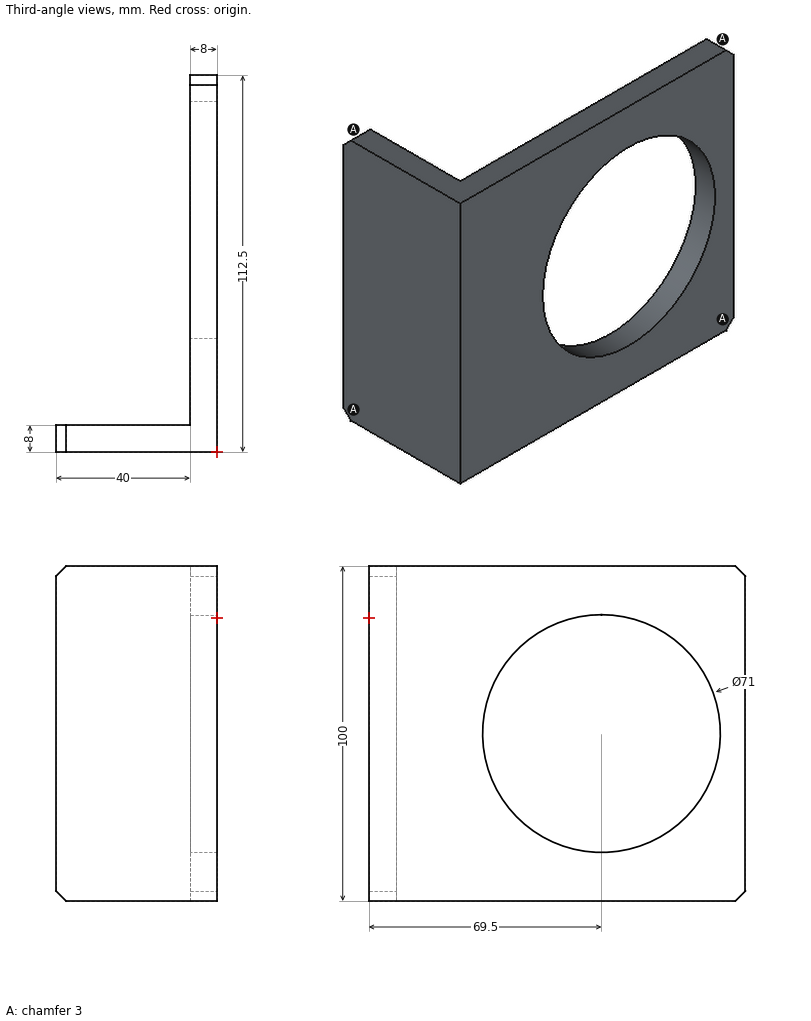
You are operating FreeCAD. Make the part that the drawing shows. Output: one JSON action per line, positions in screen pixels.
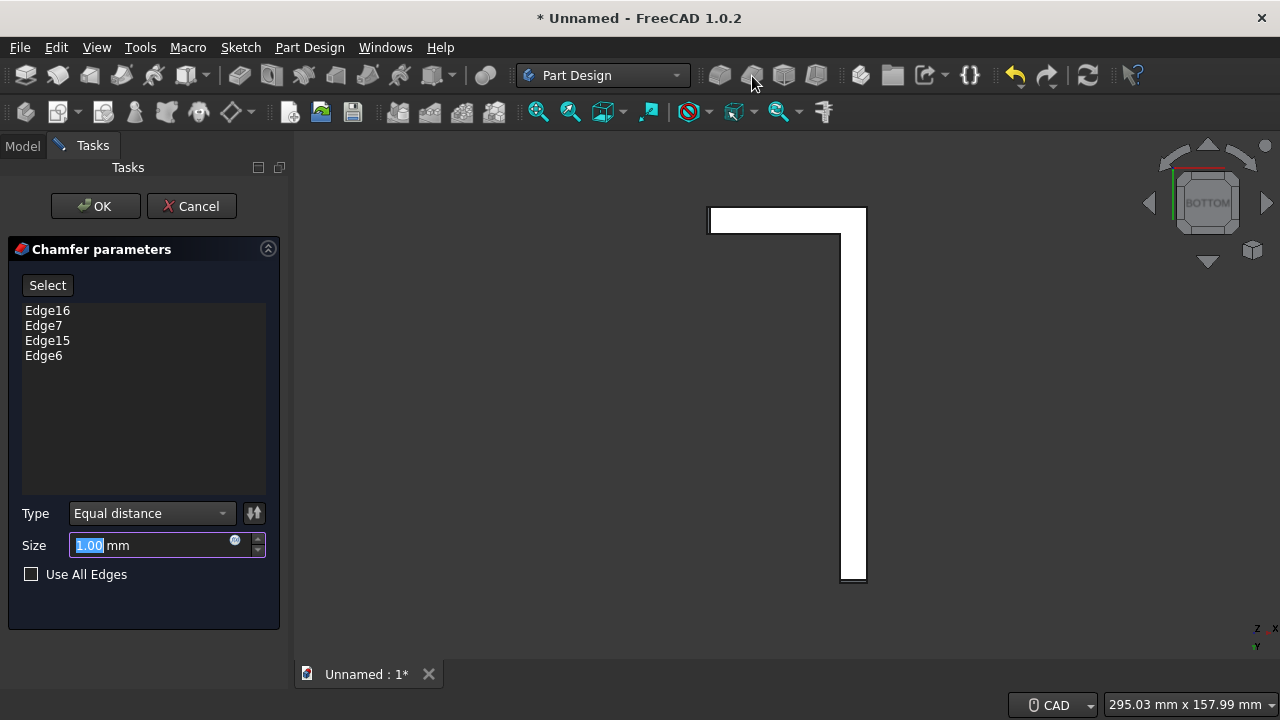
{"action": "type", "text": "3"}
{"action": "key", "text": "Tab"}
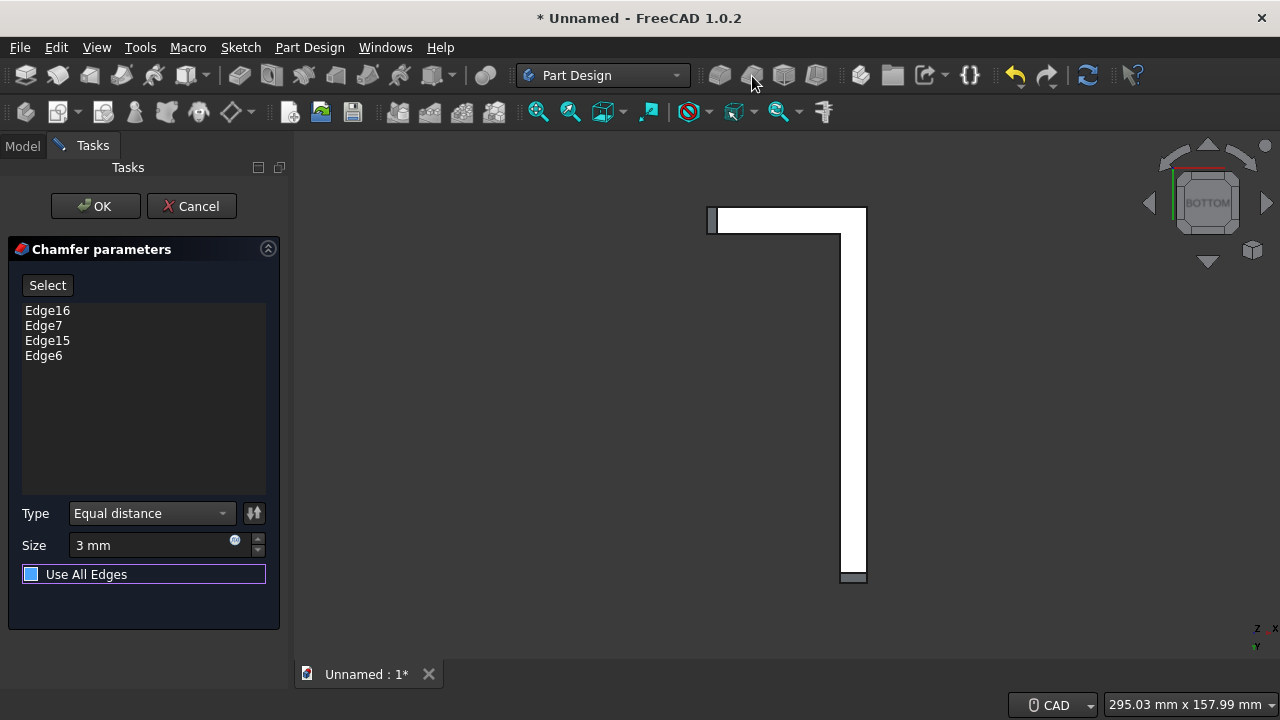
{"action": "left_click", "coordinate": [96, 206]}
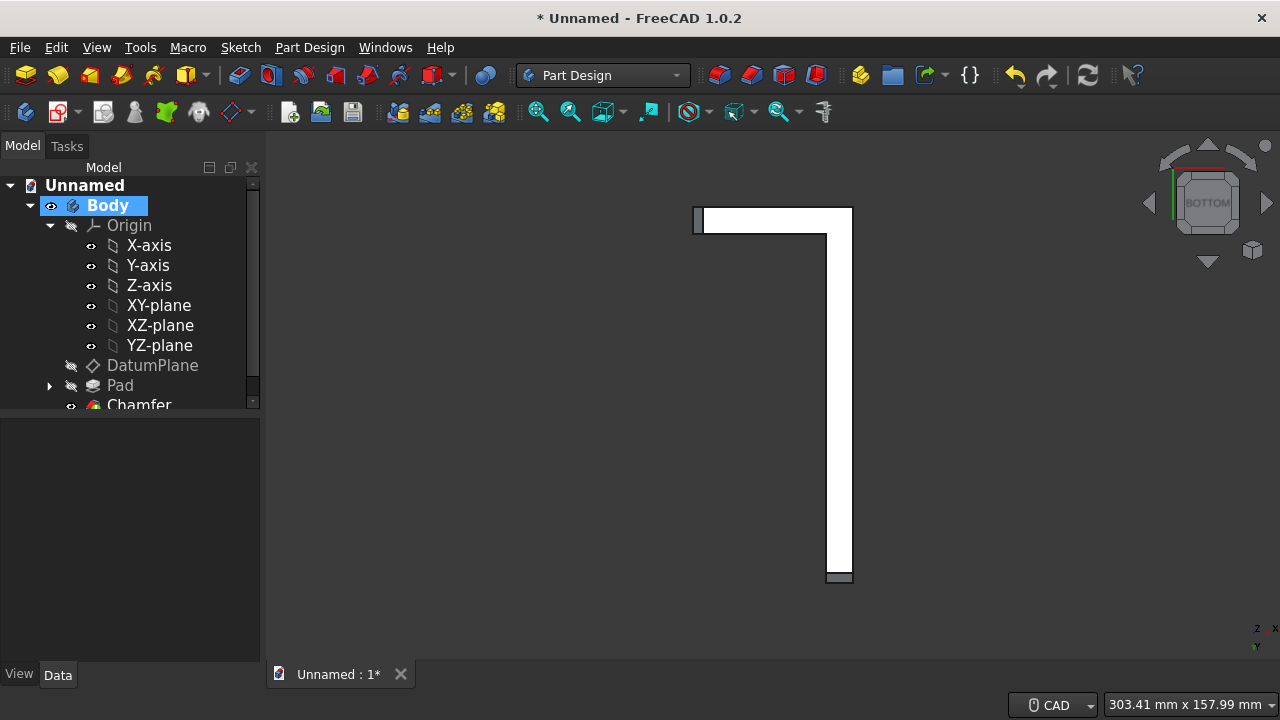
{"action": "key", "text": "6"}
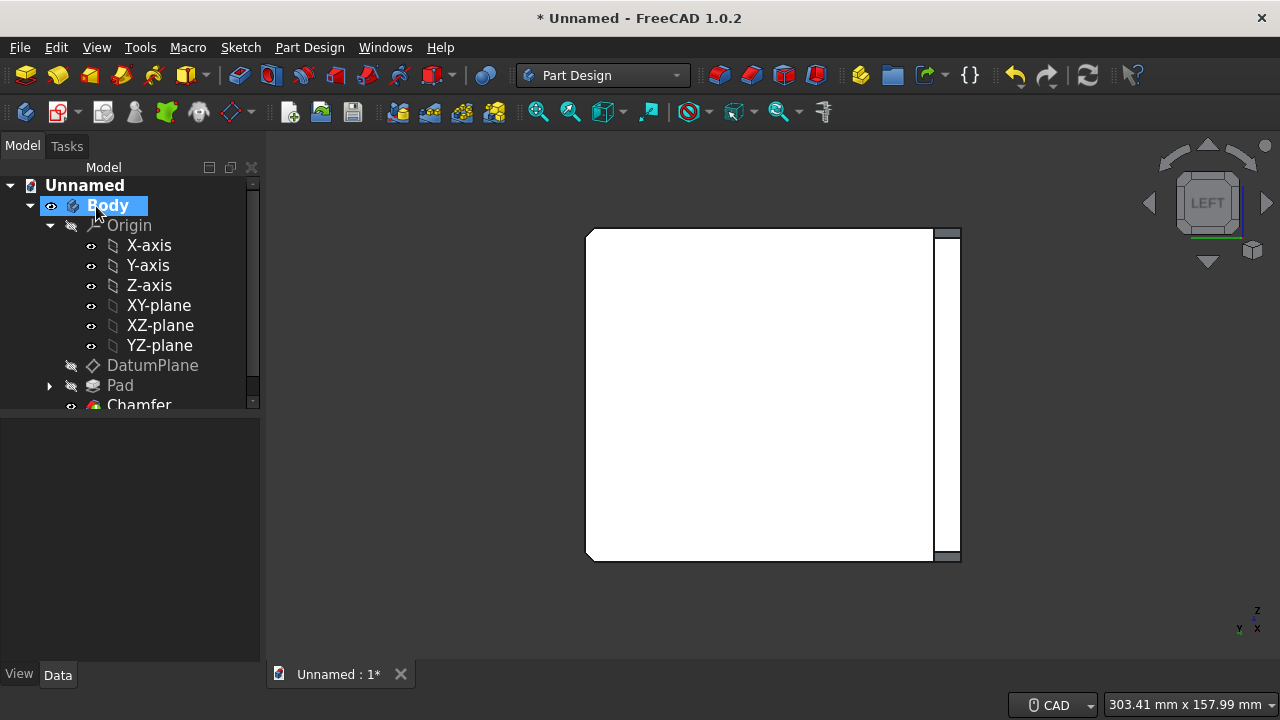
{"action": "left_click", "coordinate": [760, 394]}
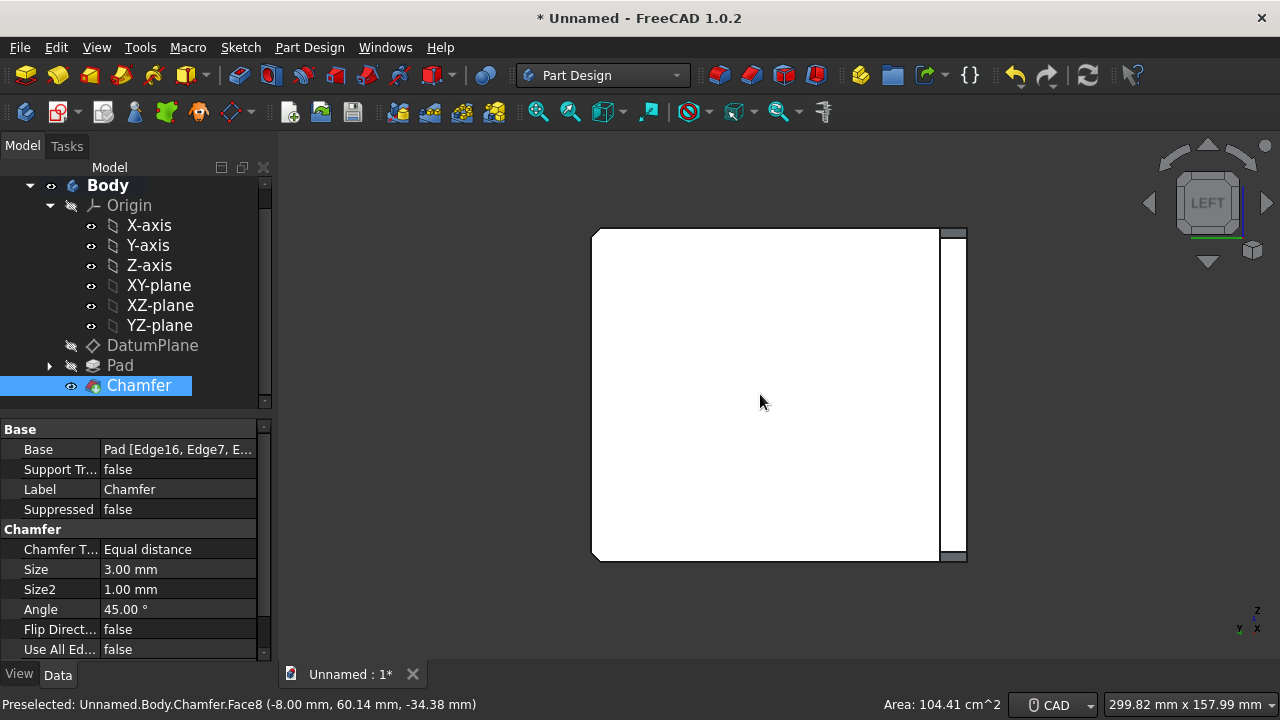
{"action": "left_click", "coordinate": [58, 112]}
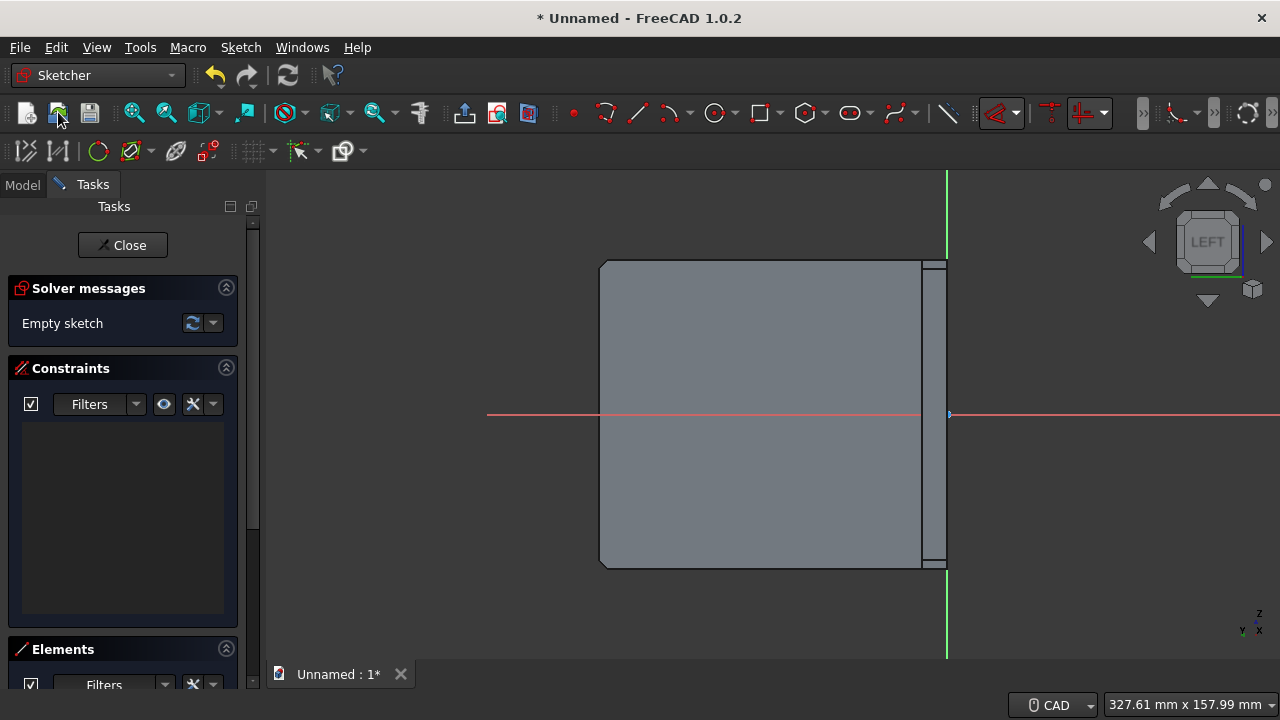
{"action": "left_click", "coordinate": [530, 114]}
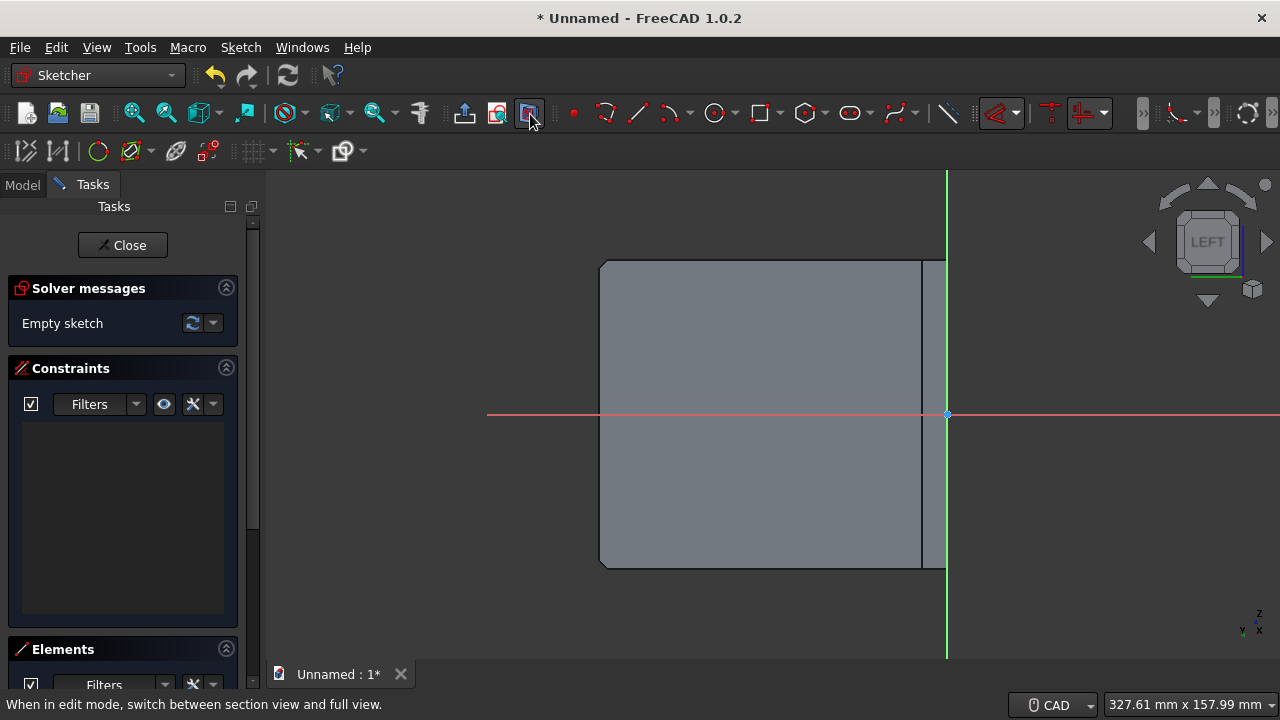
{"action": "scroll", "coordinate": [947, 414], "scroll_direction": "up", "scroll_amount": 2}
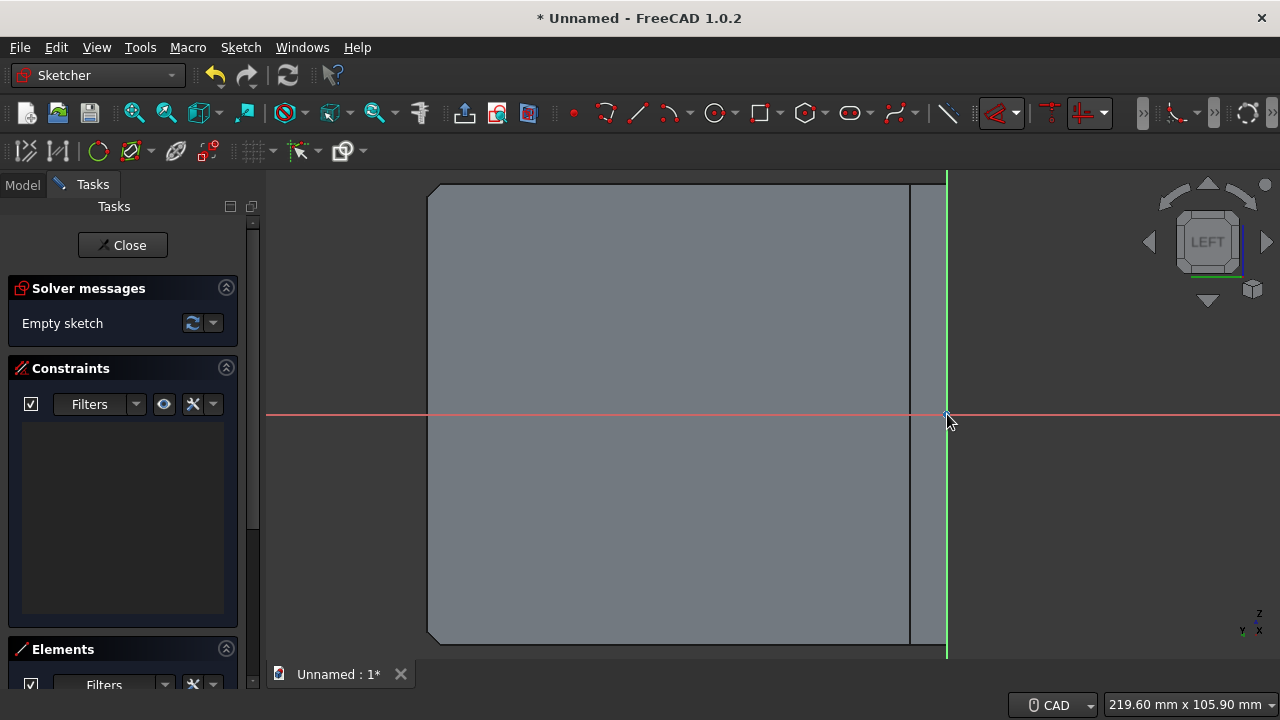
{"action": "left_click", "coordinate": [716, 114]}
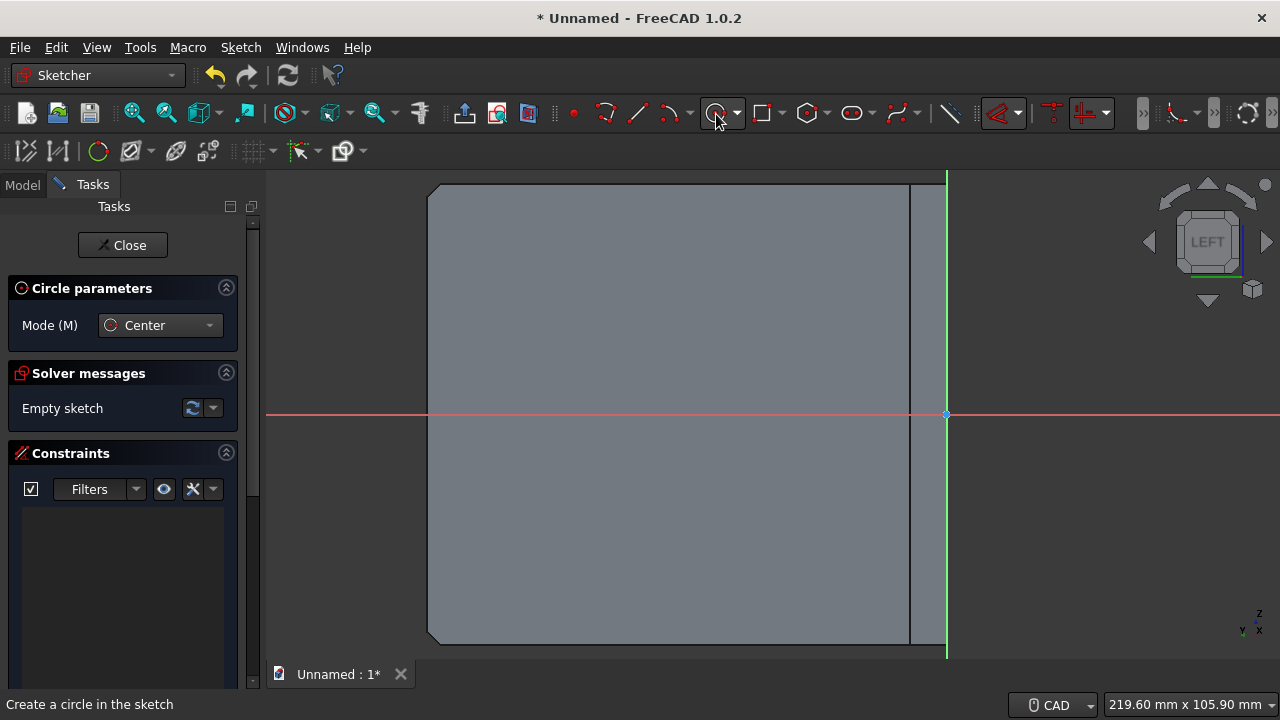
{"action": "left_click", "coordinate": [626, 414]}
{"action": "left_click", "coordinate": [742, 299]}
{"action": "key", "text": "Escape"}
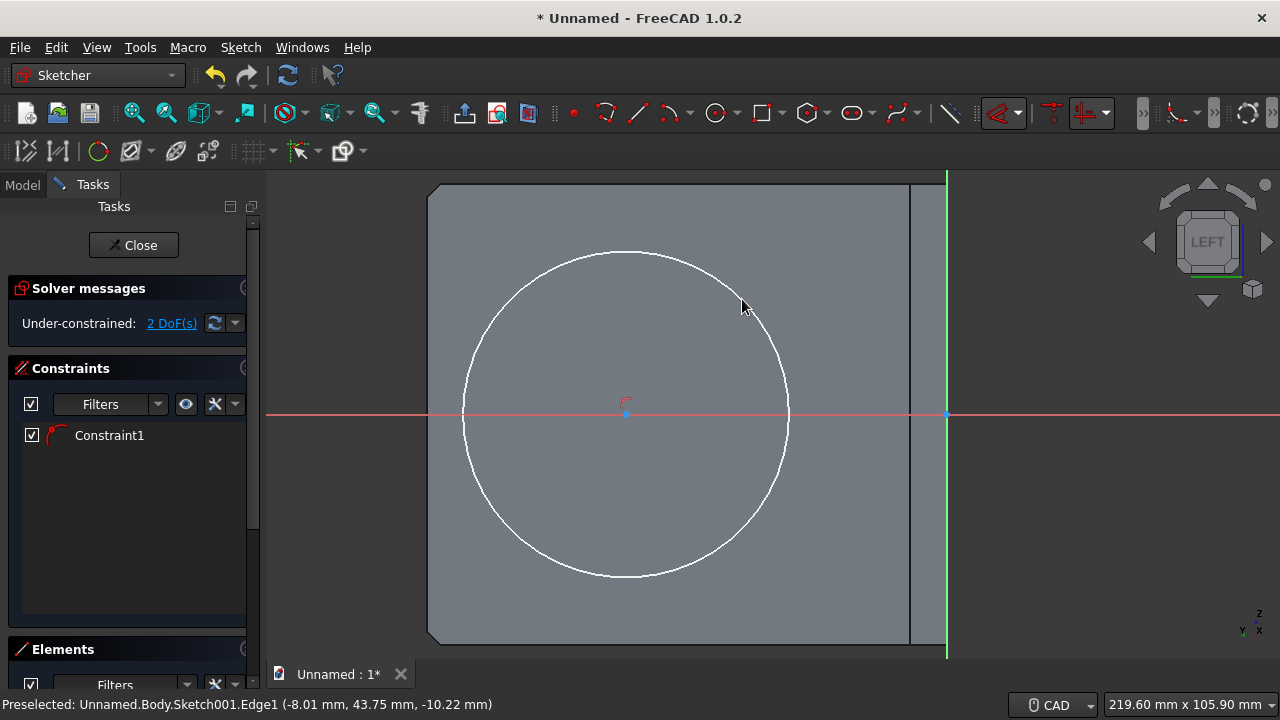
{"action": "left_click", "coordinate": [741, 299]}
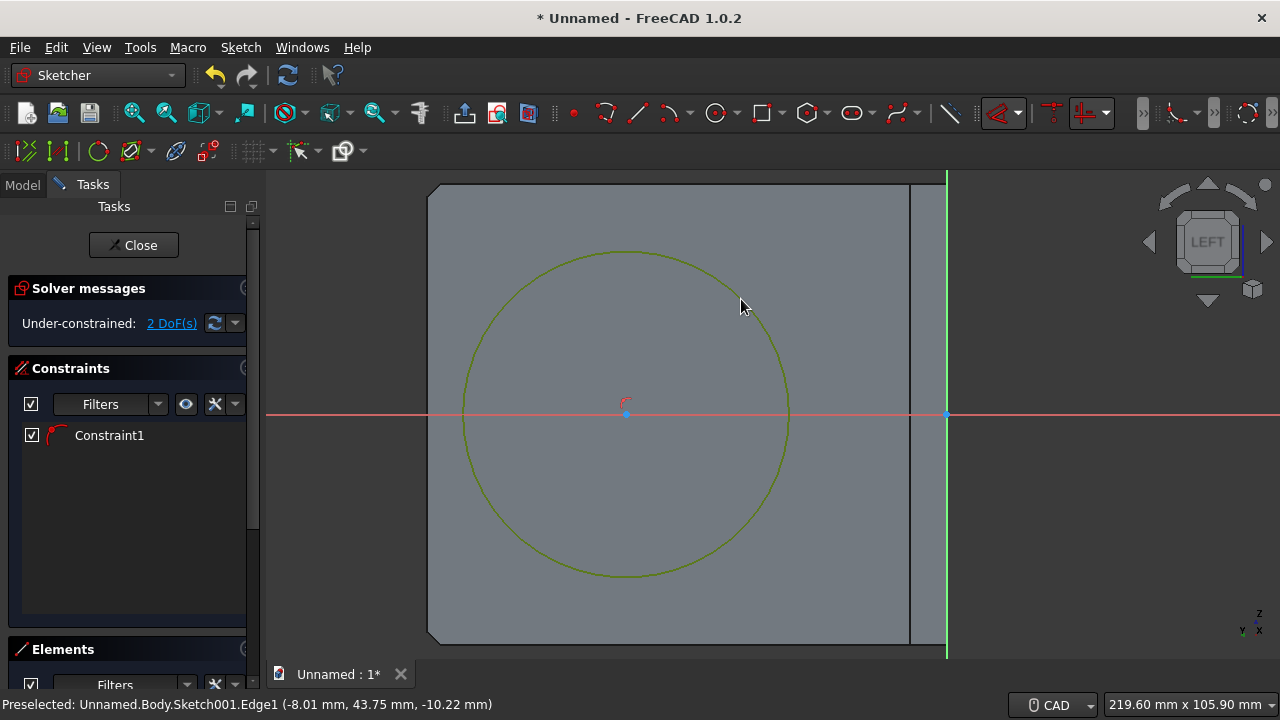
{"action": "key", "text": "k o"}